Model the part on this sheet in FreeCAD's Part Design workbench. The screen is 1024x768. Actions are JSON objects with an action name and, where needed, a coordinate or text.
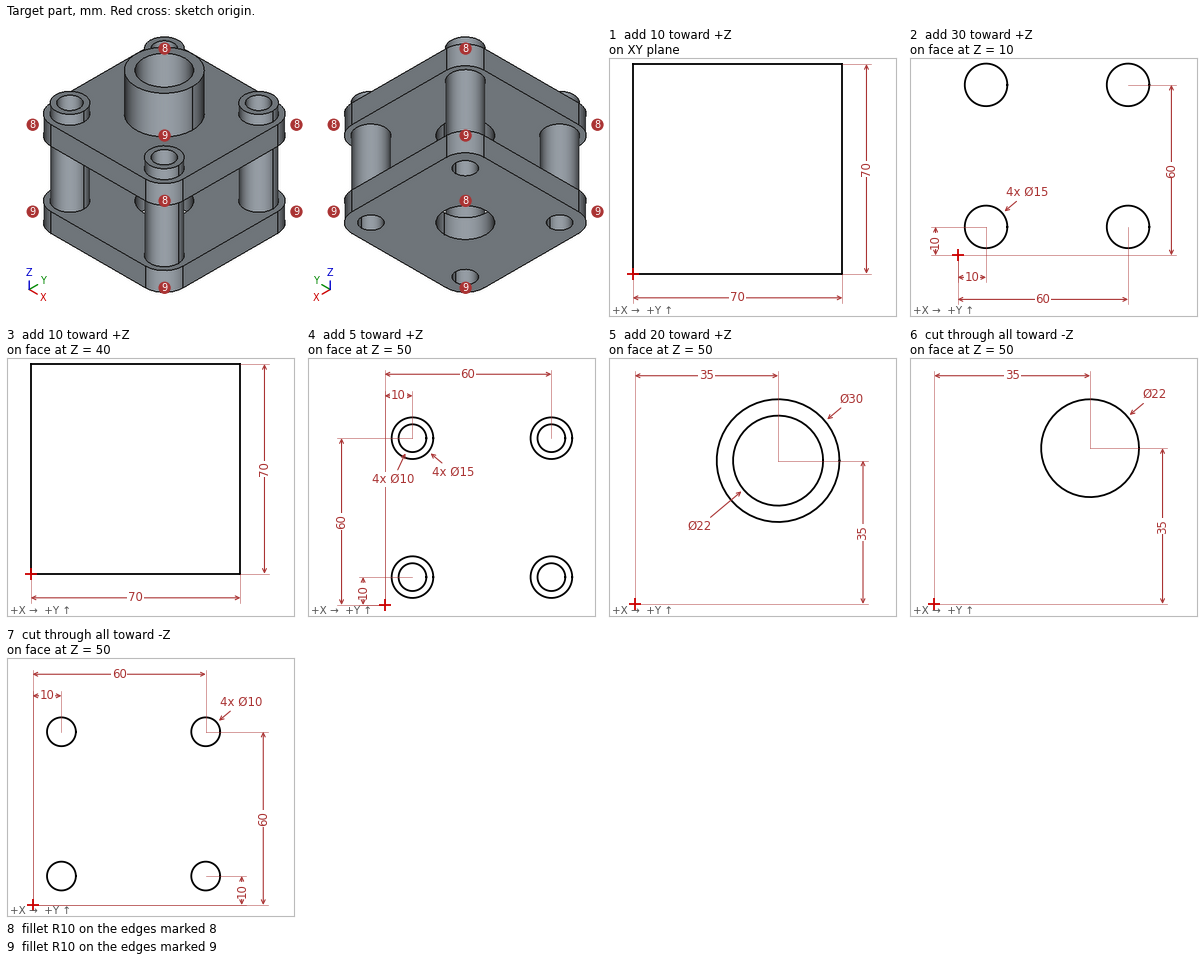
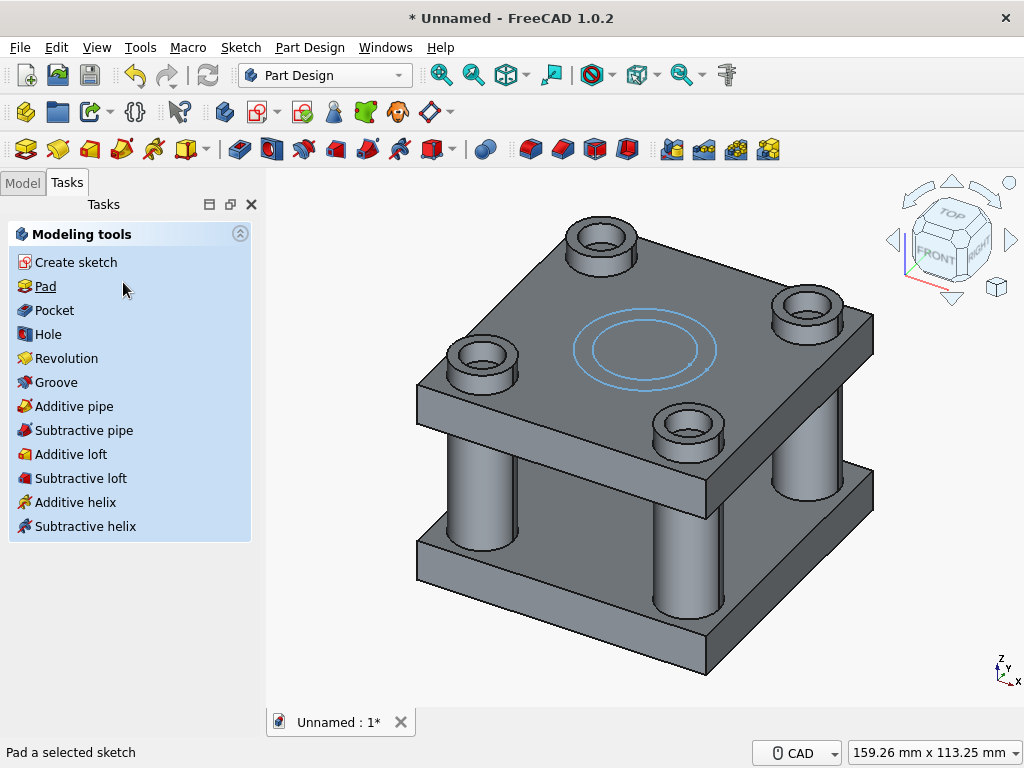
{"action": "left_click", "coordinate": [26, 150]}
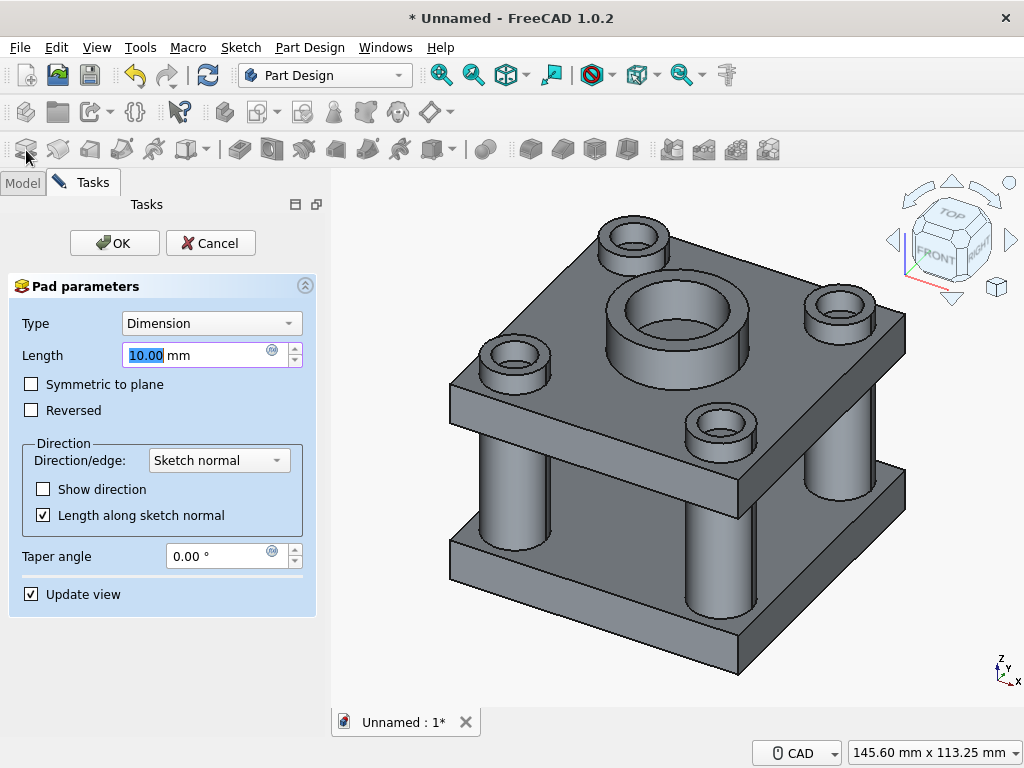
{"action": "type", "text": "20"}
{"action": "key", "text": "Tab"}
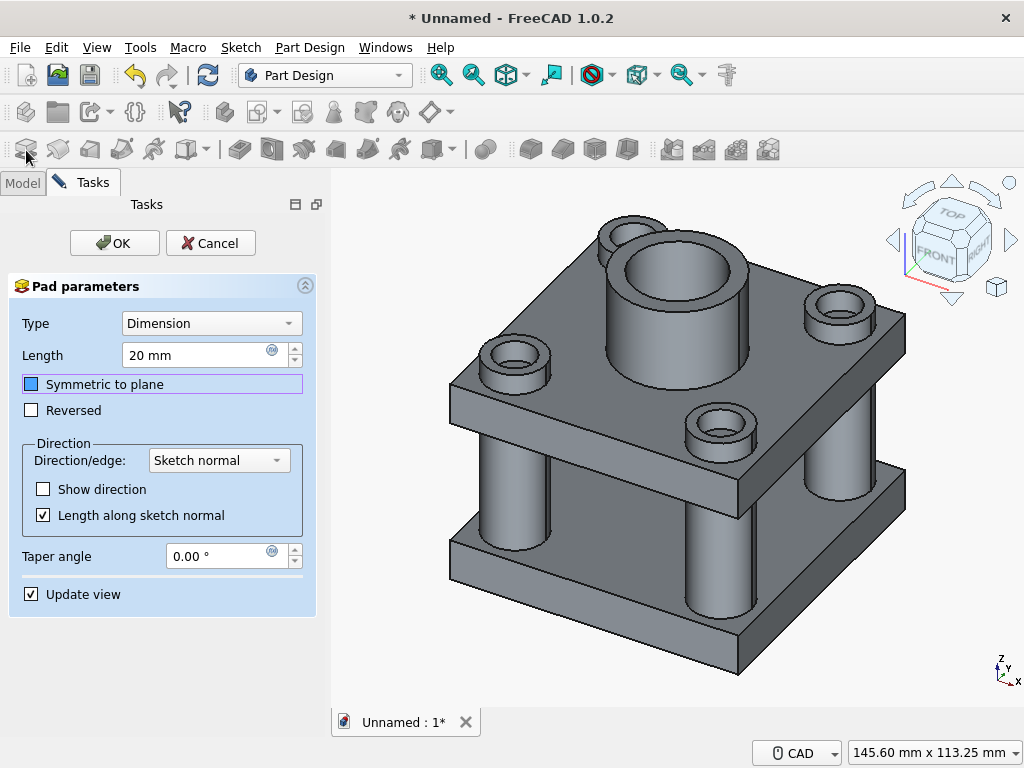
{"action": "left_click", "coordinate": [115, 243]}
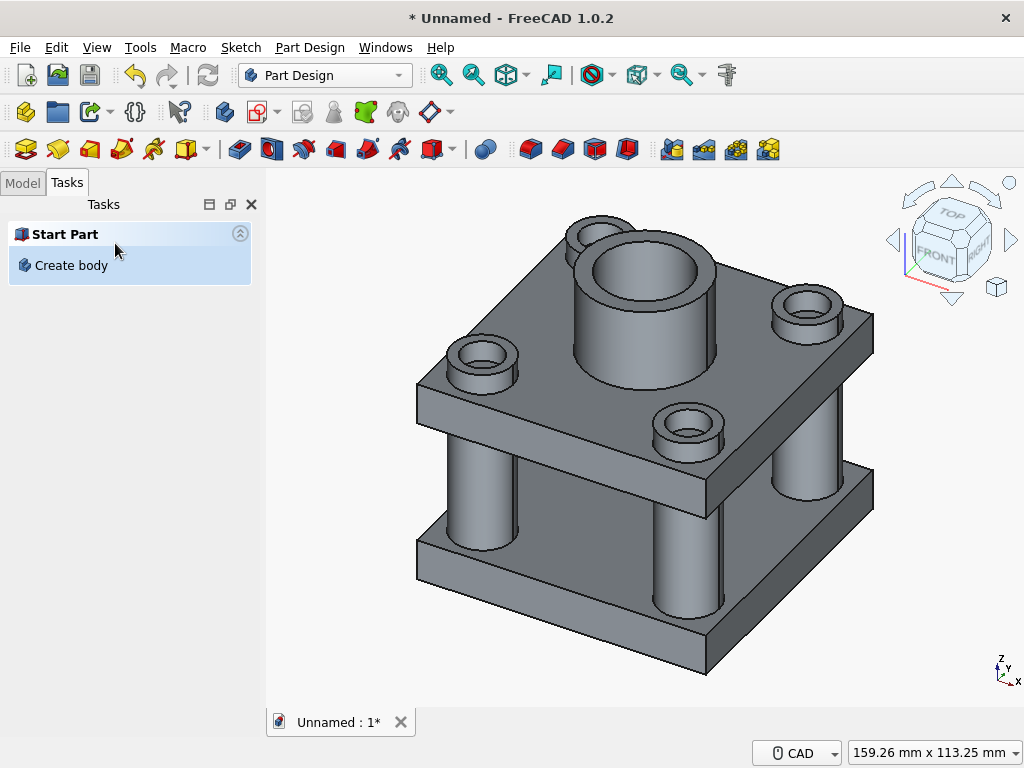
{"action": "key", "text": "v f"}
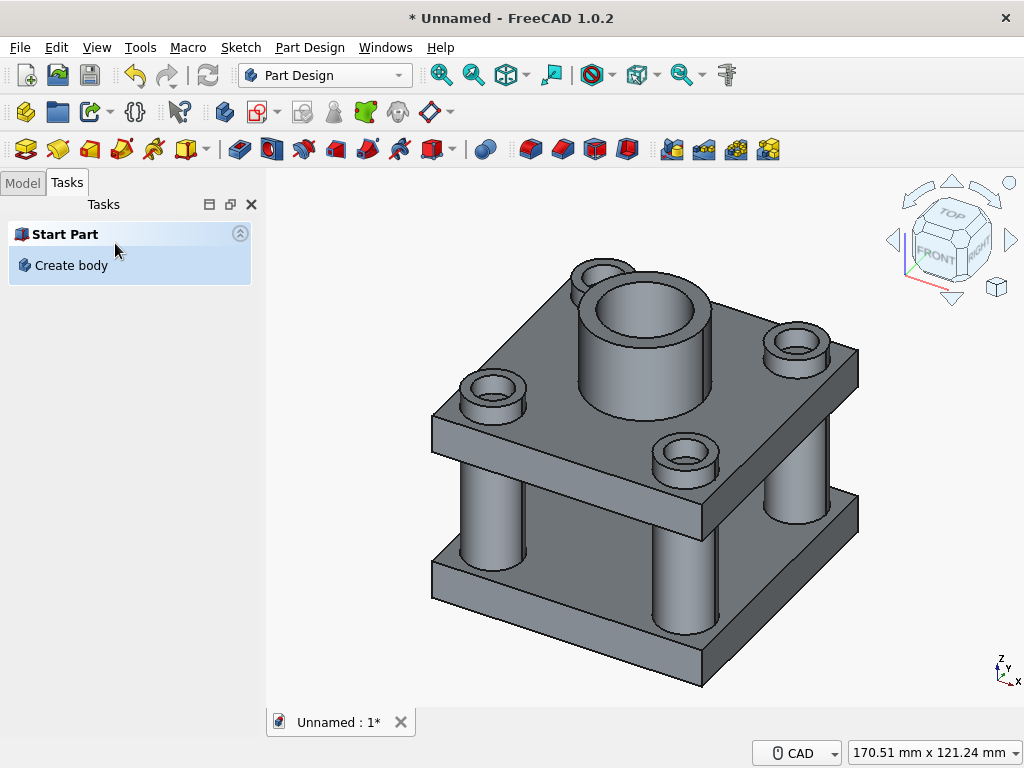
{"action": "left_click", "coordinate": [744, 385]}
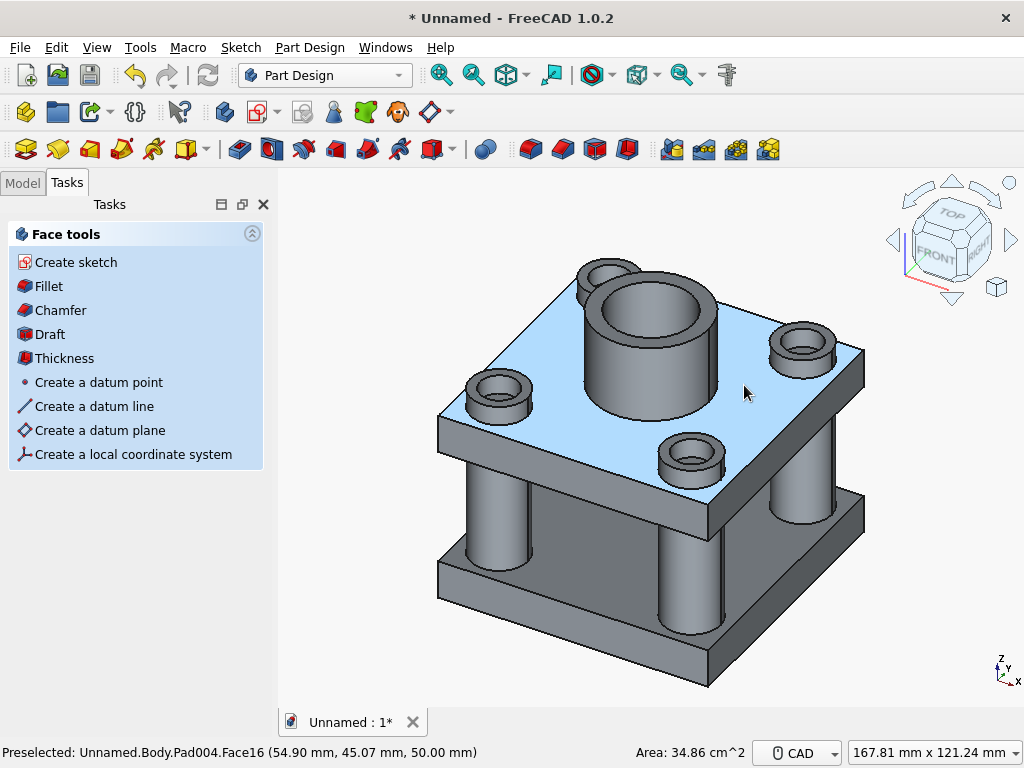
{"action": "left_click", "coordinate": [258, 112]}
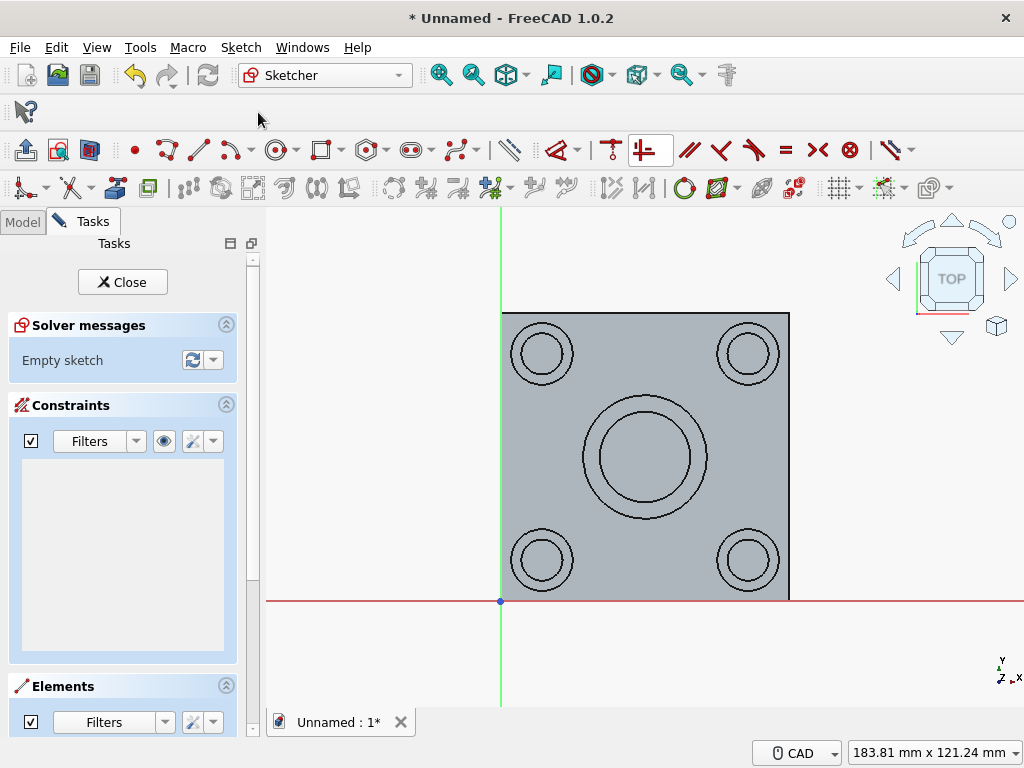
{"action": "left_click", "coordinate": [90, 150]}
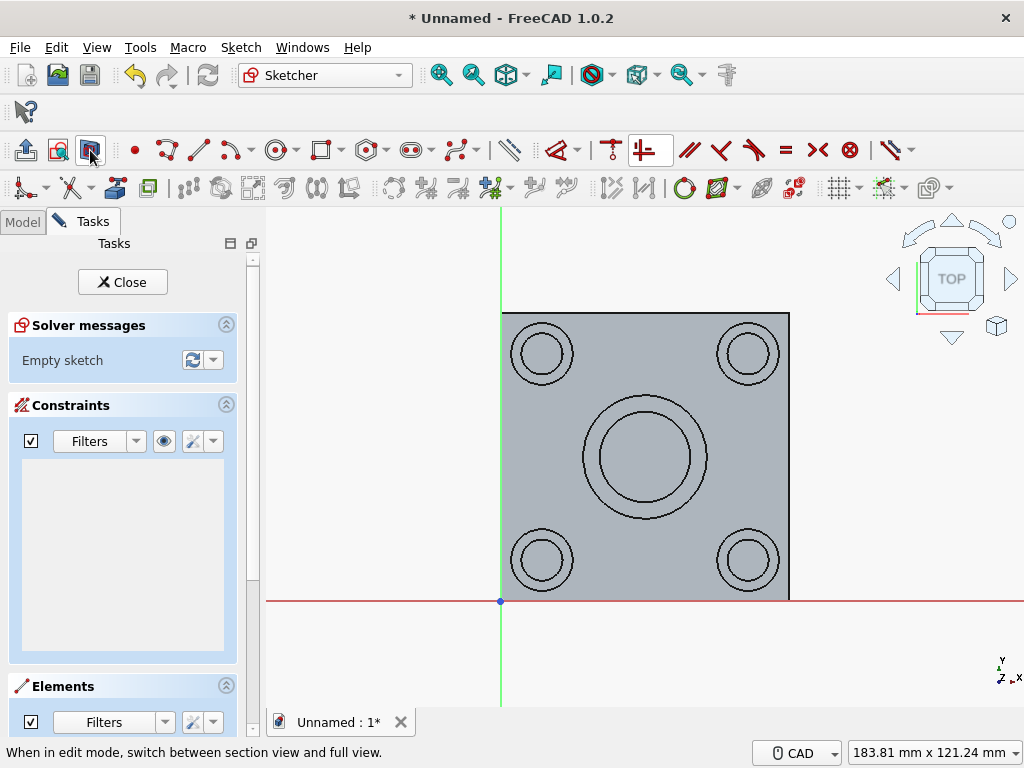
{"action": "scroll", "coordinate": [619, 567], "scroll_direction": "up", "scroll_amount": 3}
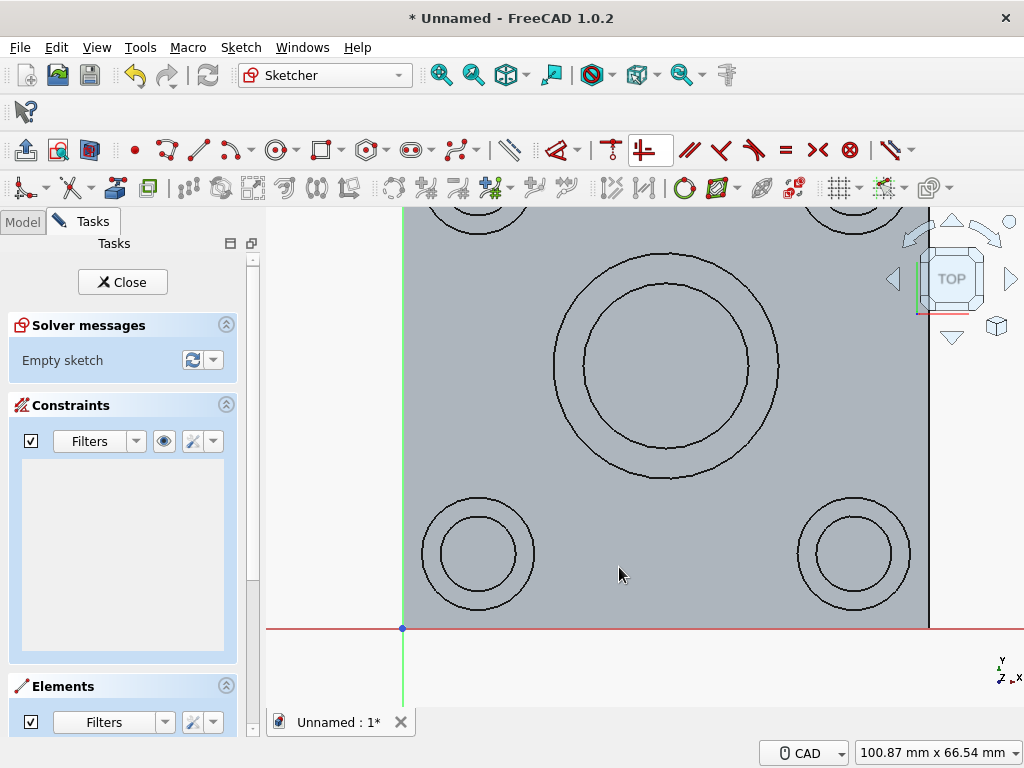
{"action": "left_click", "coordinate": [276, 150]}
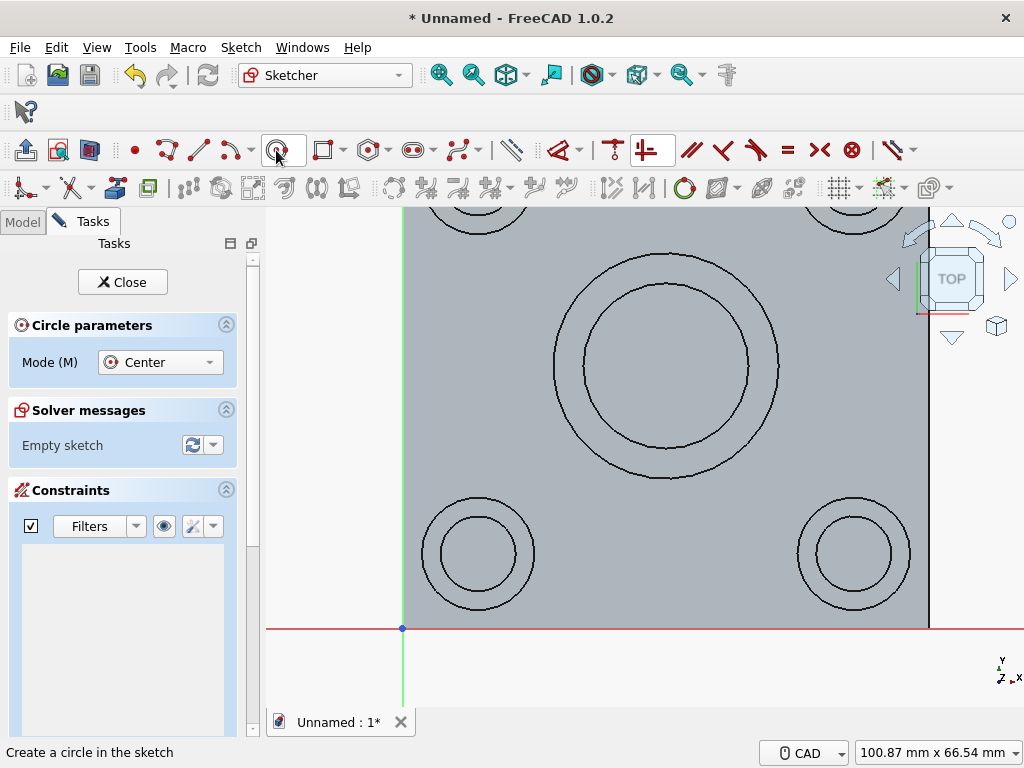
{"action": "left_click", "coordinate": [666, 366]}
{"action": "left_click", "coordinate": [724, 308]}
{"action": "key", "text": "Escape"}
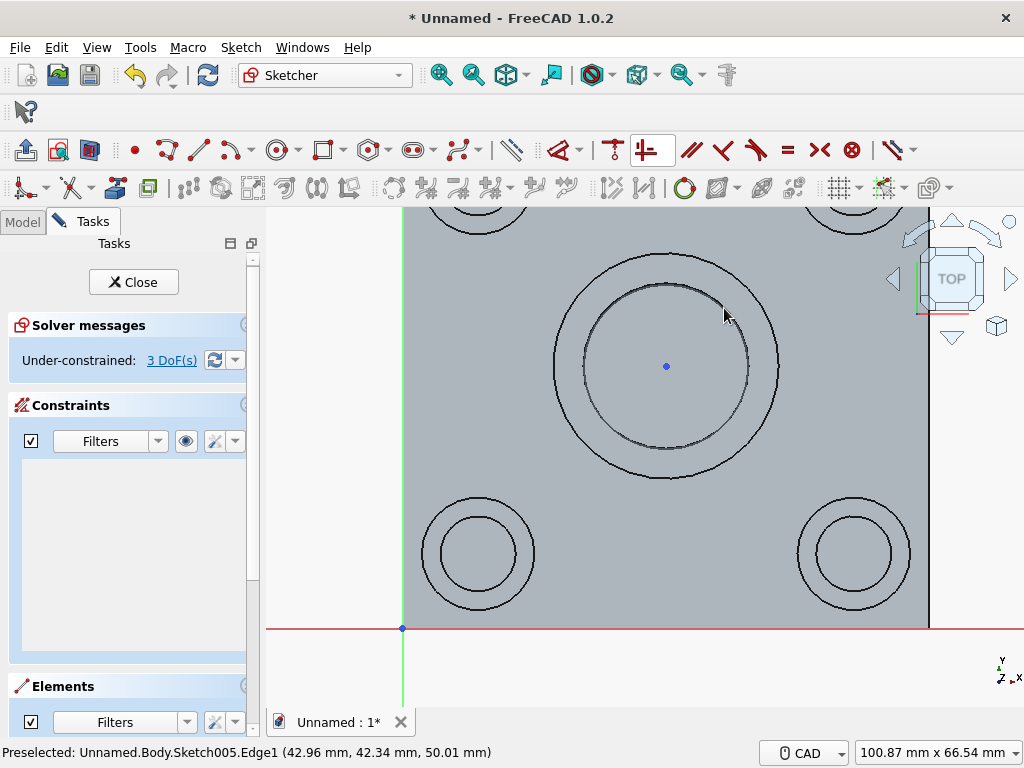
{"action": "key", "text": "d"}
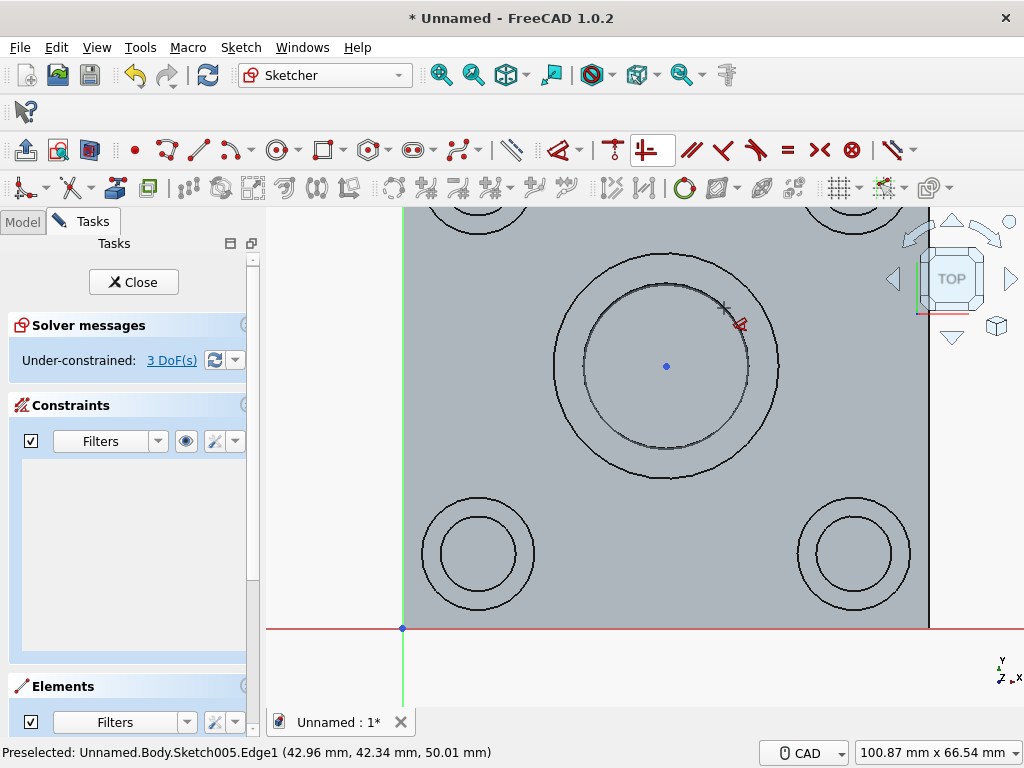
{"action": "left_click", "coordinate": [724, 309]}
{"action": "left_click", "coordinate": [747, 286]}